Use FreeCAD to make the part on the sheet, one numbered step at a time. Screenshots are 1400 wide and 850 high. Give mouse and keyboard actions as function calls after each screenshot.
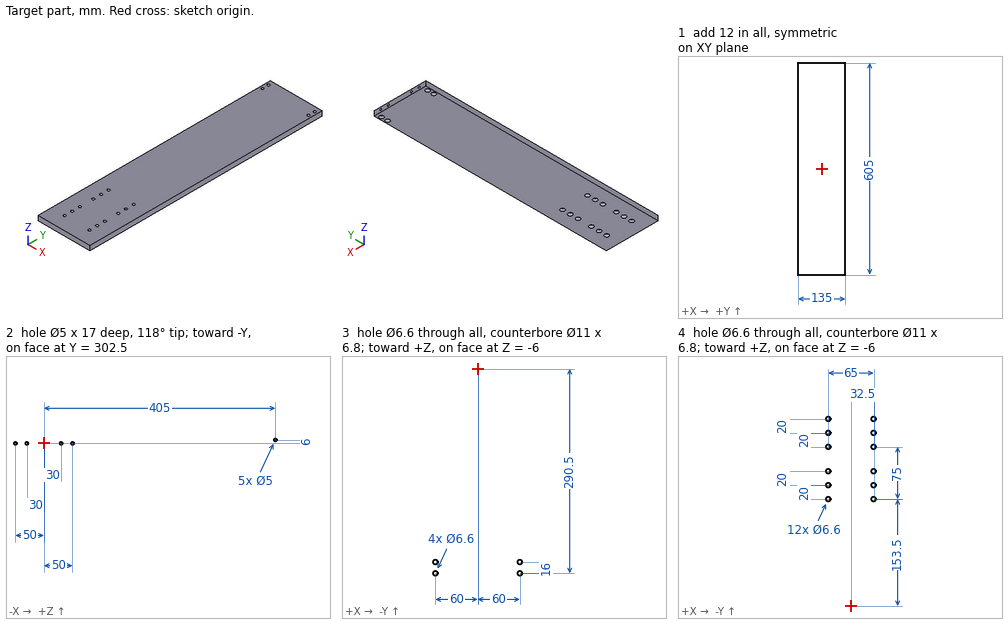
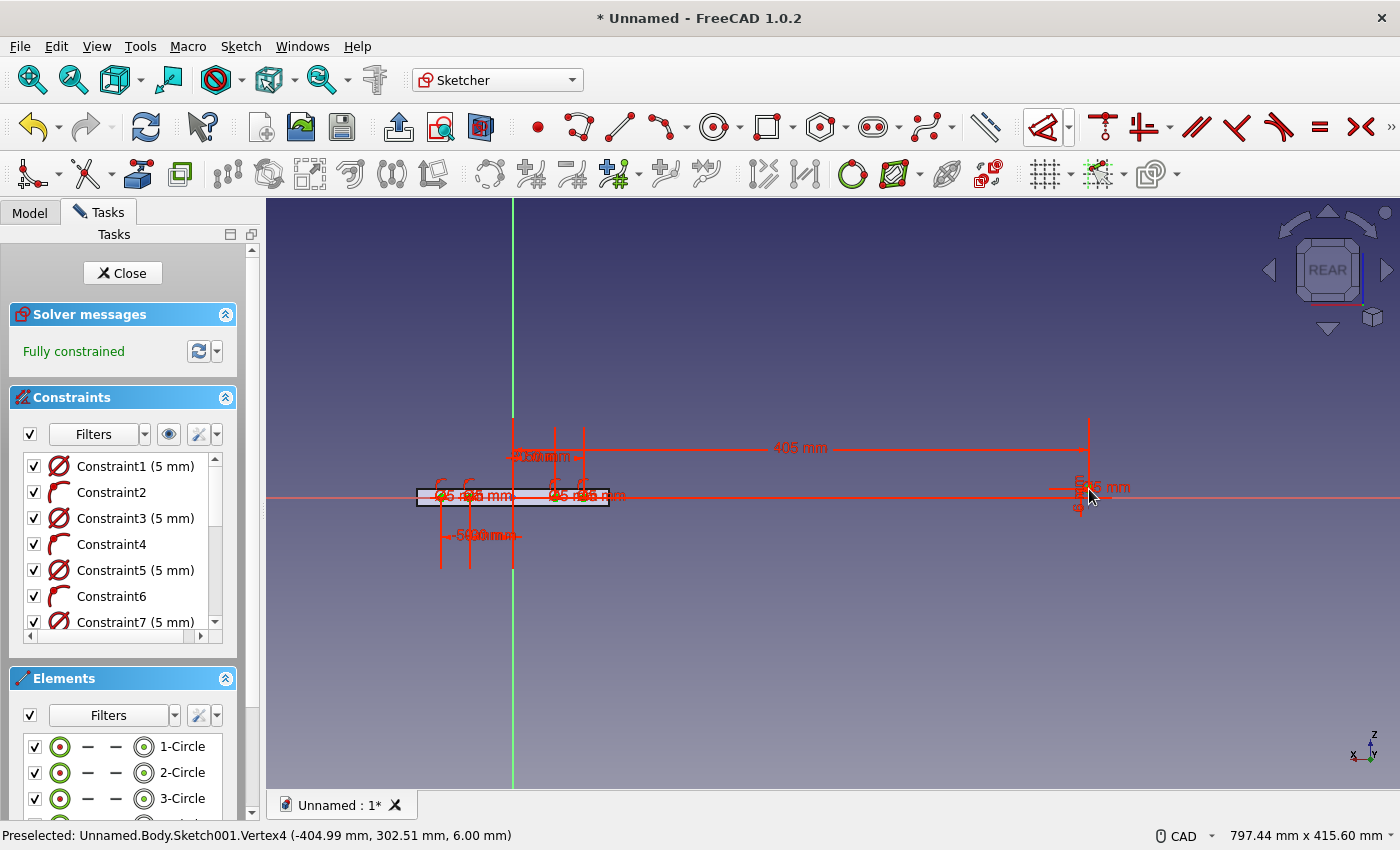
click(123, 273)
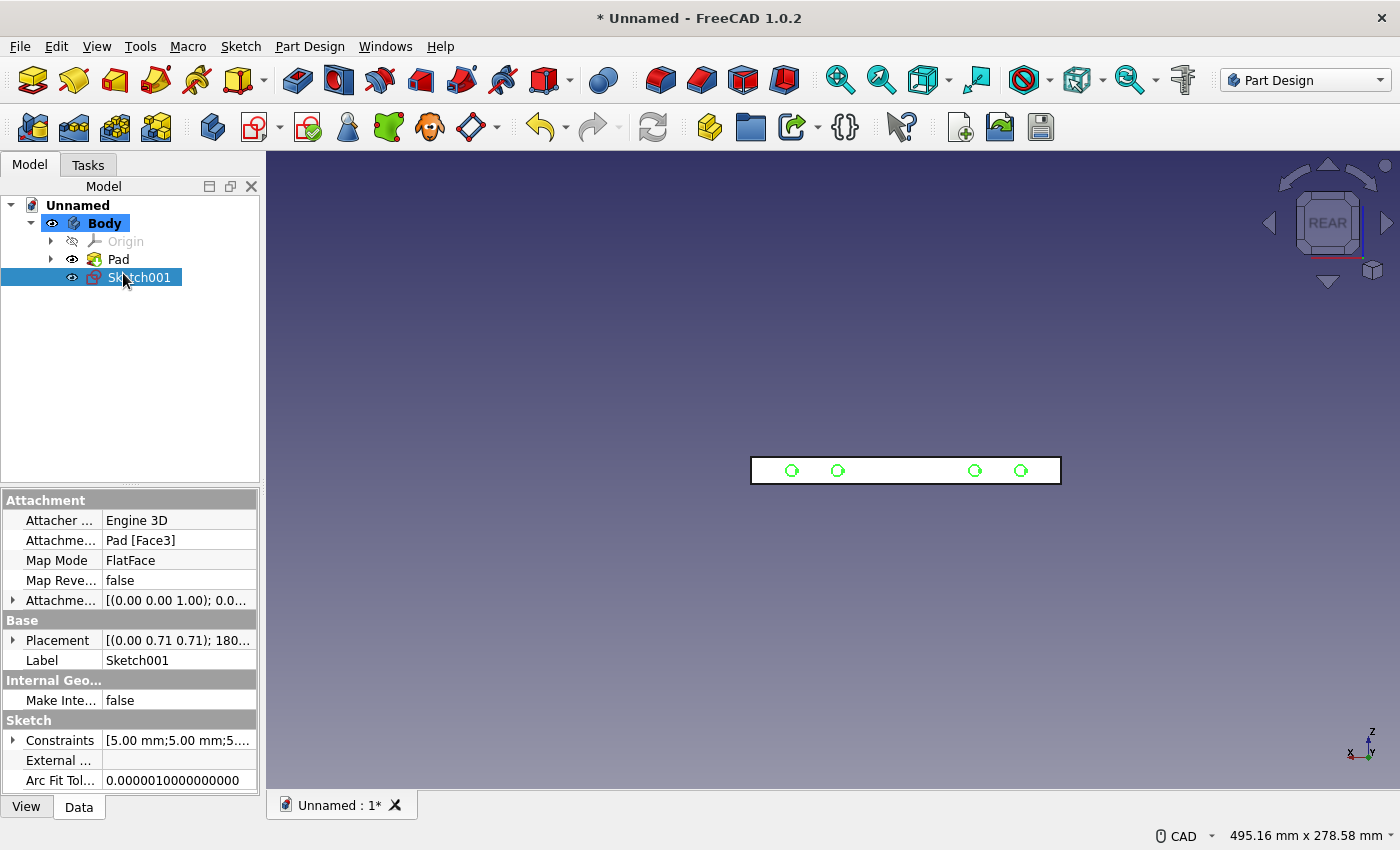
click(339, 80)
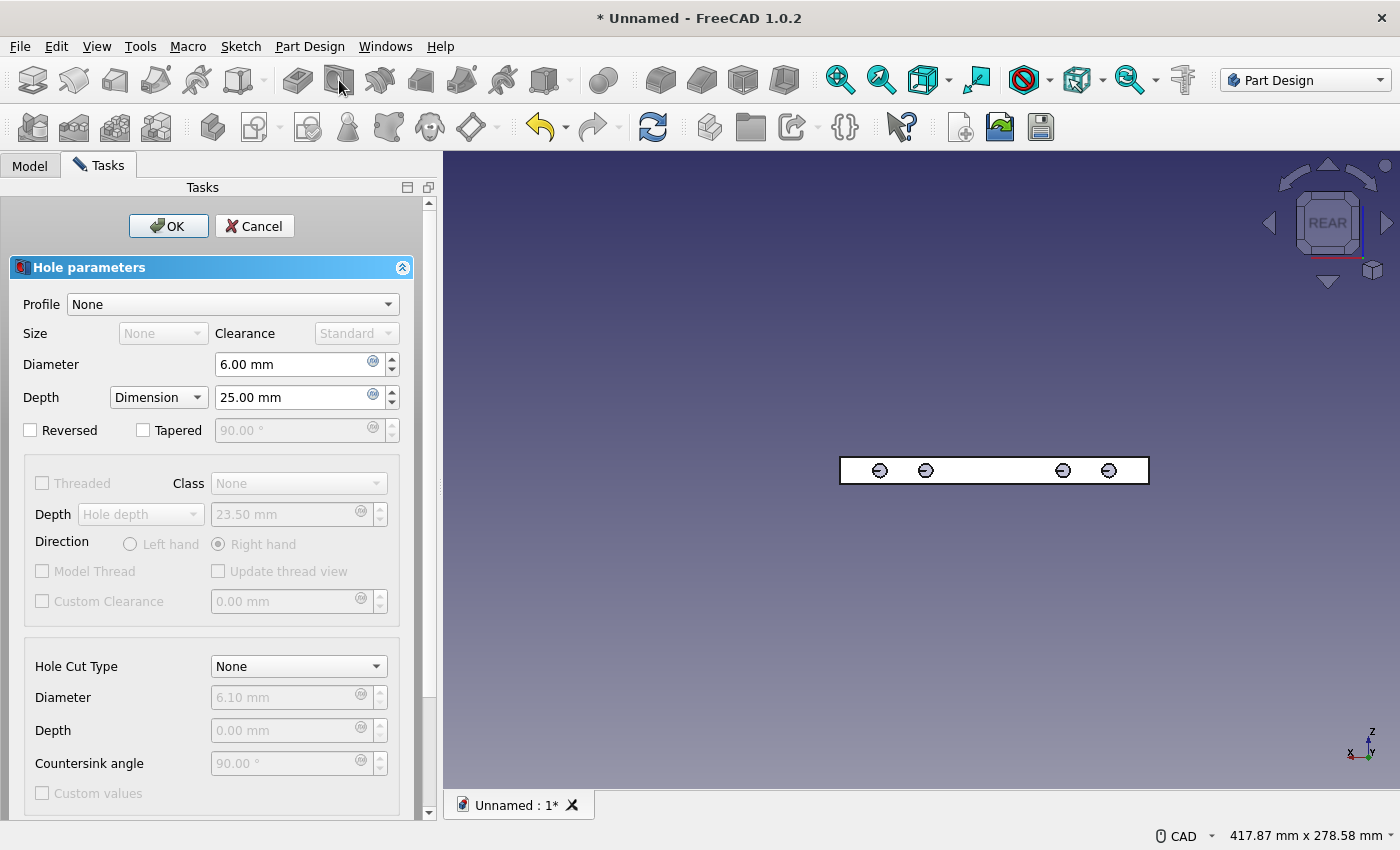
triple_click(300, 364)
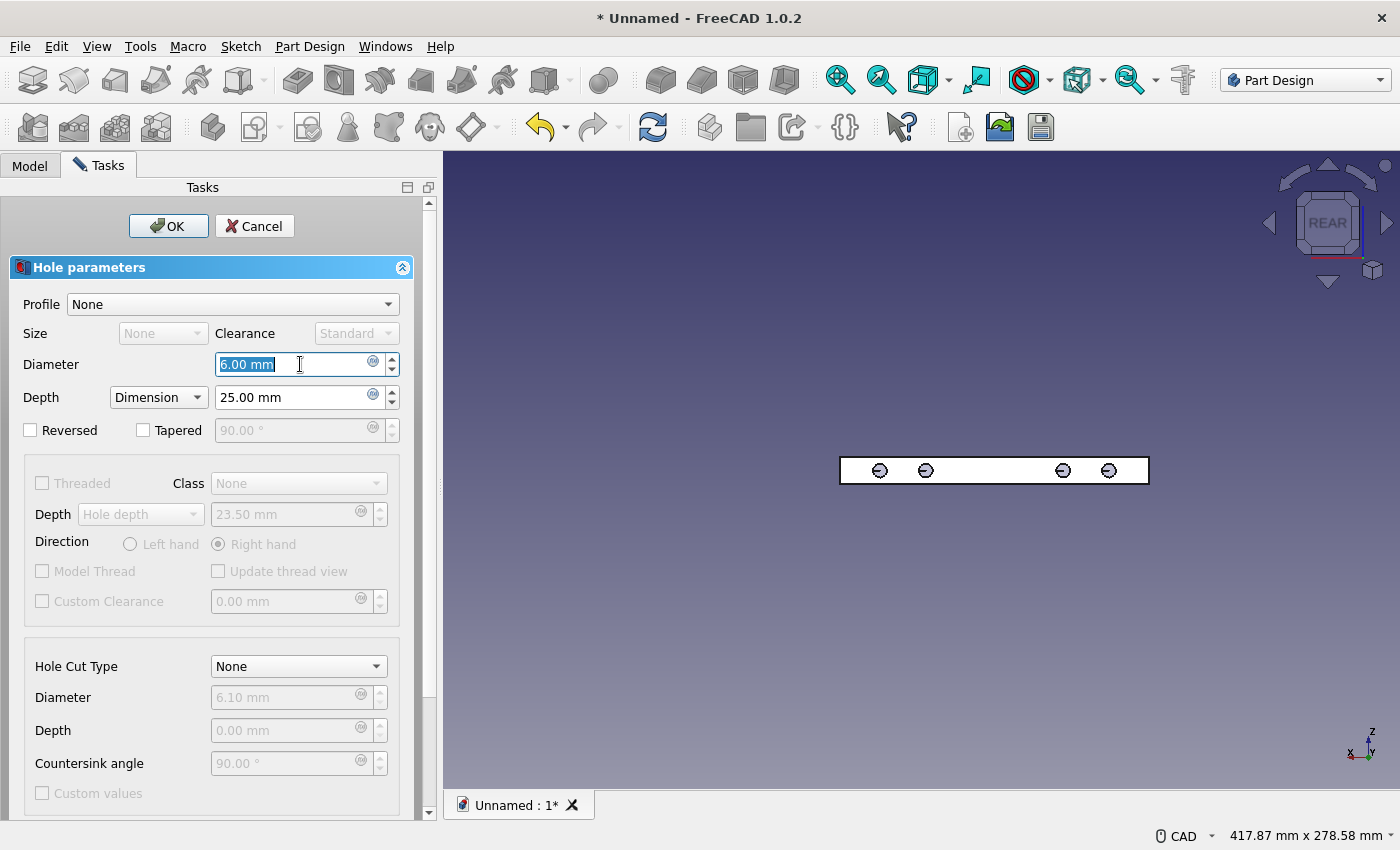
text(5)
key(Tab)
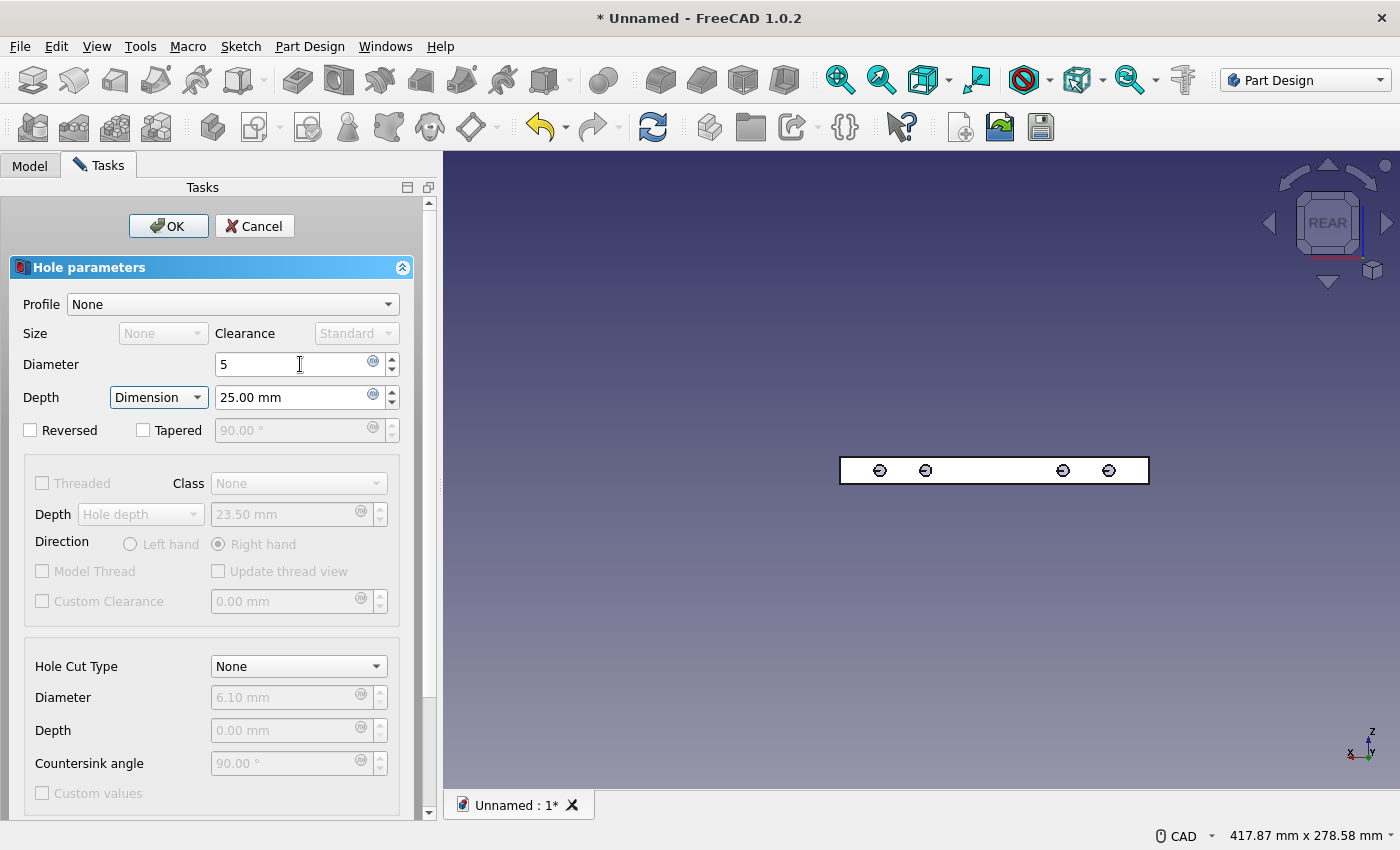
triple_click(300, 398)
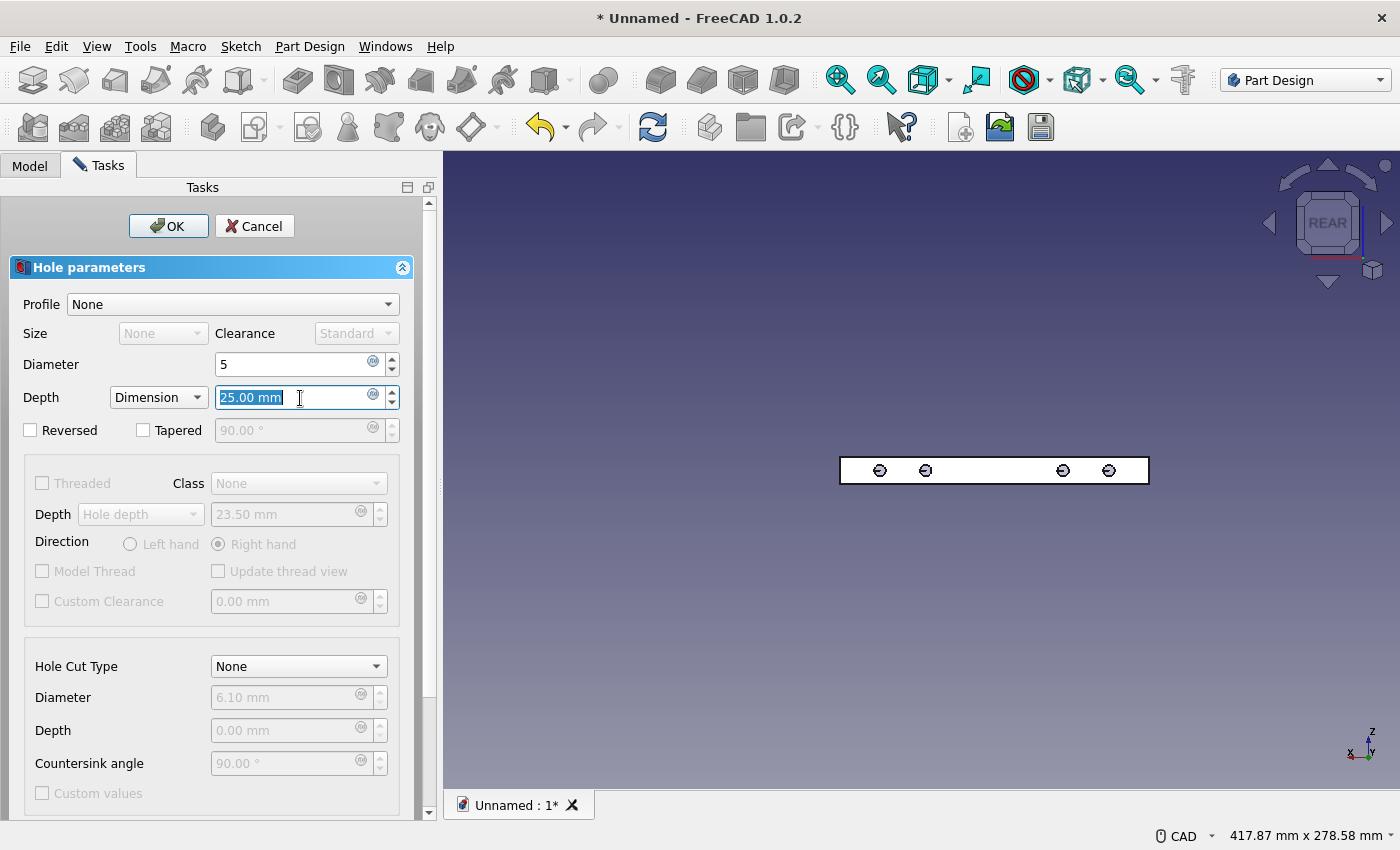
text(17)
key(Tab)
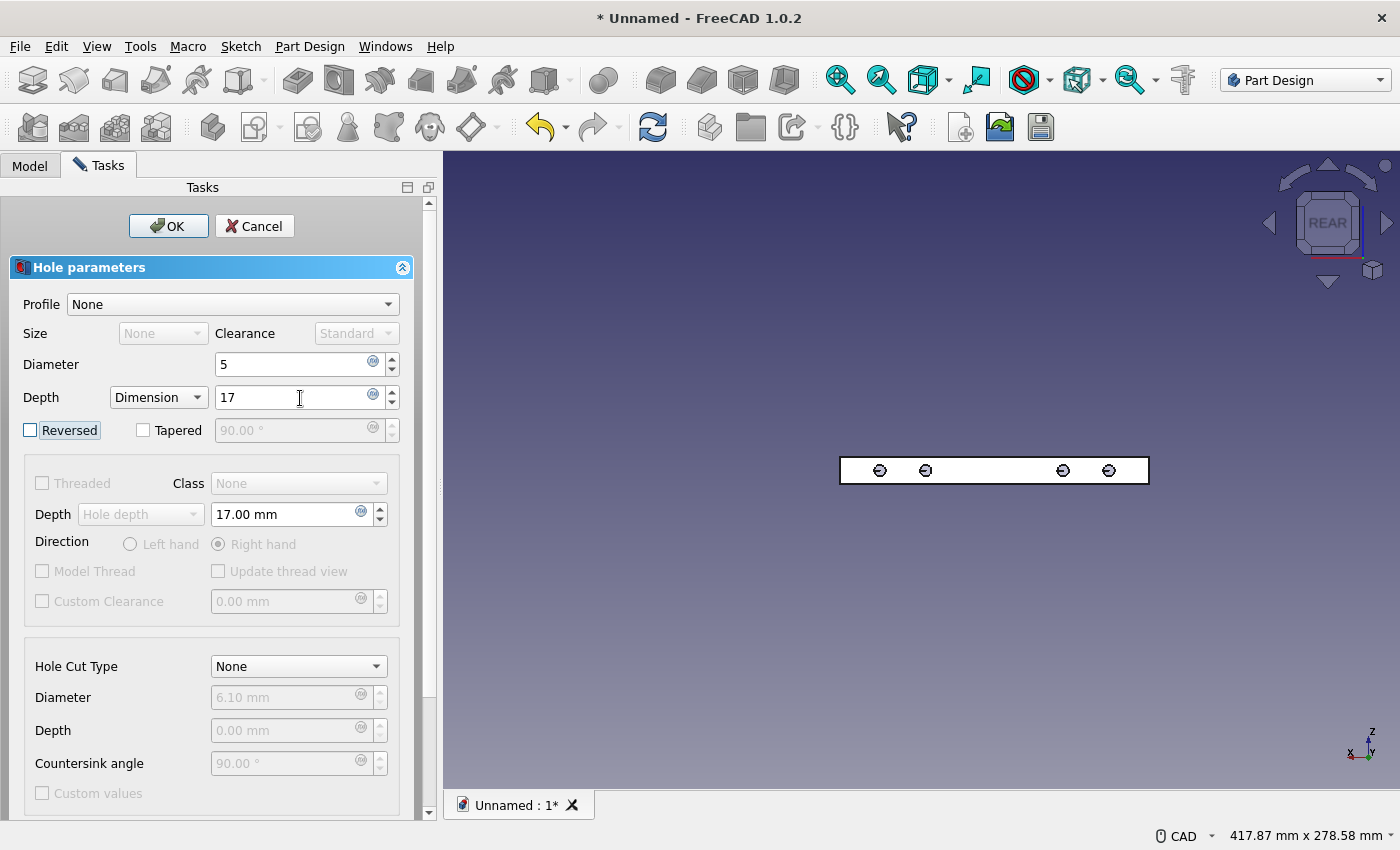
click(169, 226)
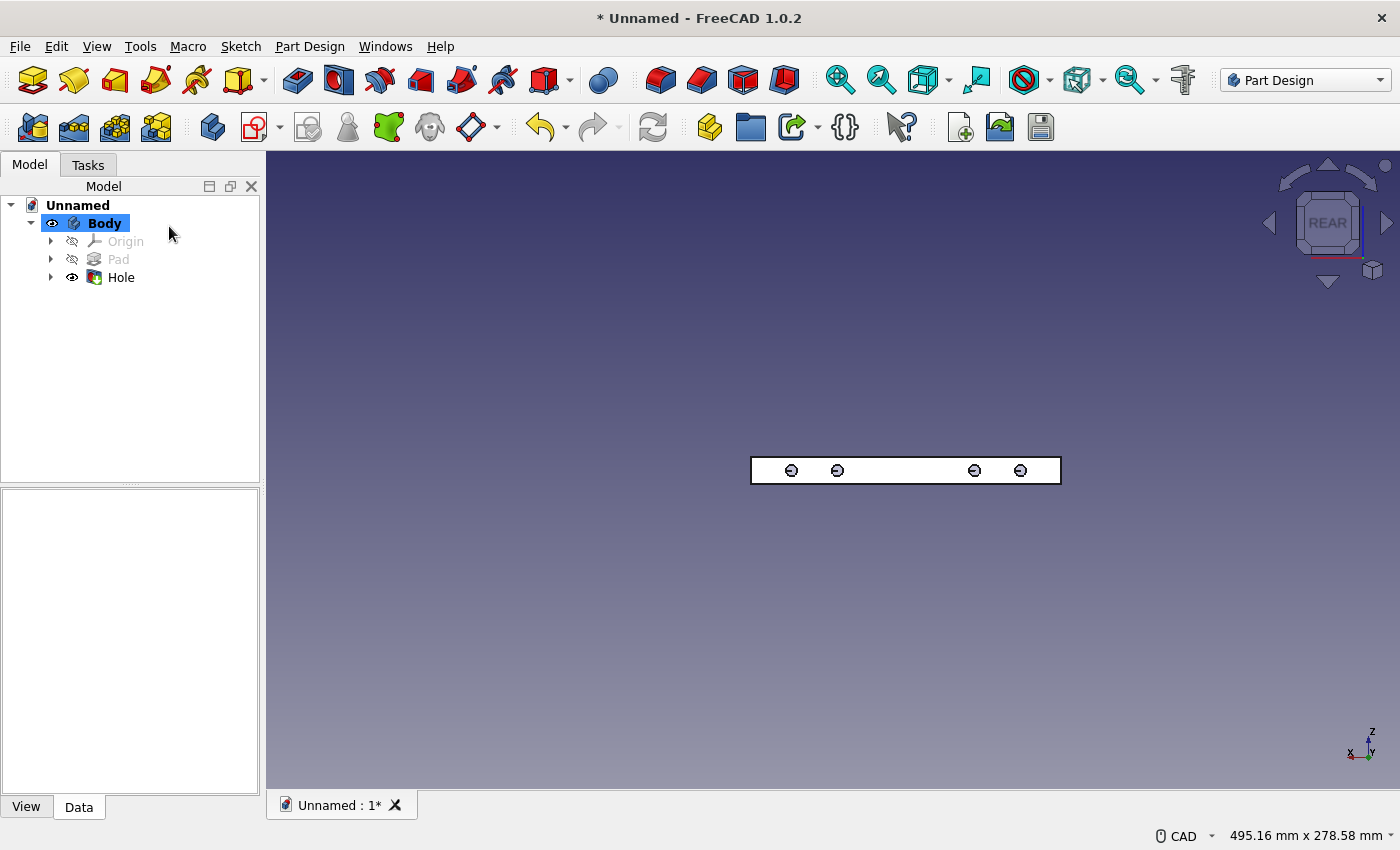
click(841, 80)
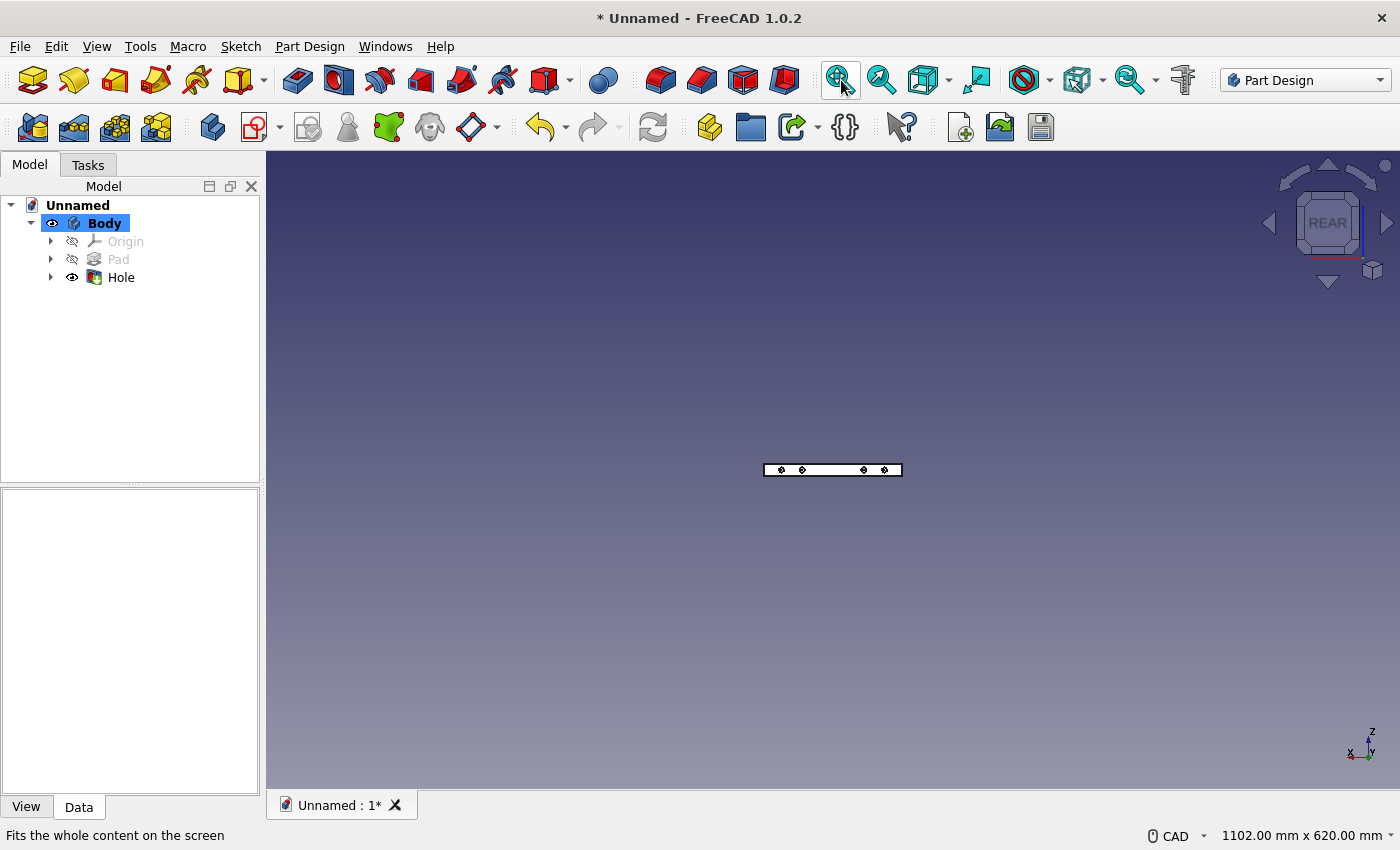
key(5)